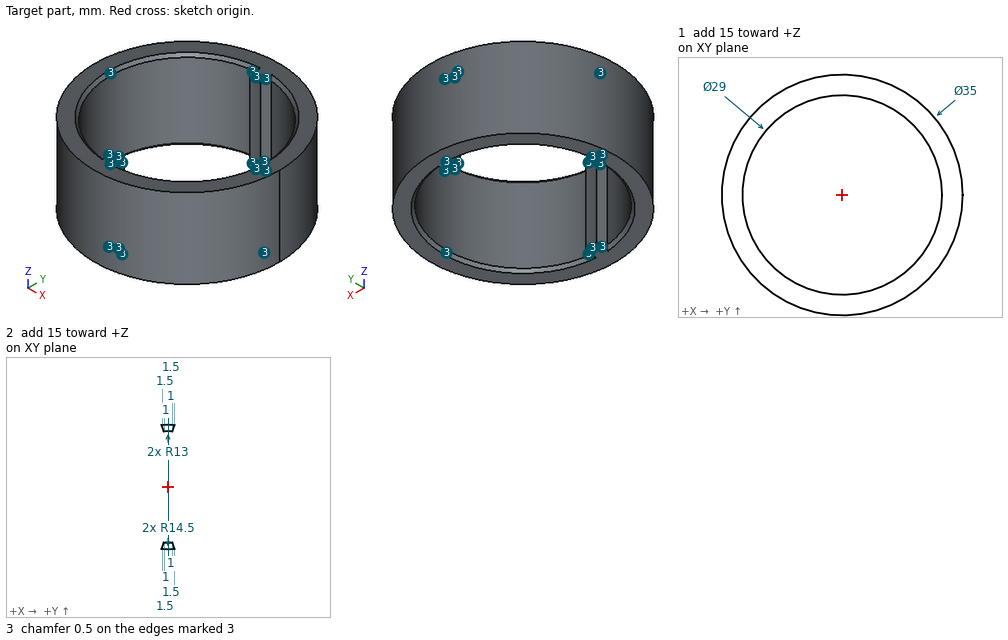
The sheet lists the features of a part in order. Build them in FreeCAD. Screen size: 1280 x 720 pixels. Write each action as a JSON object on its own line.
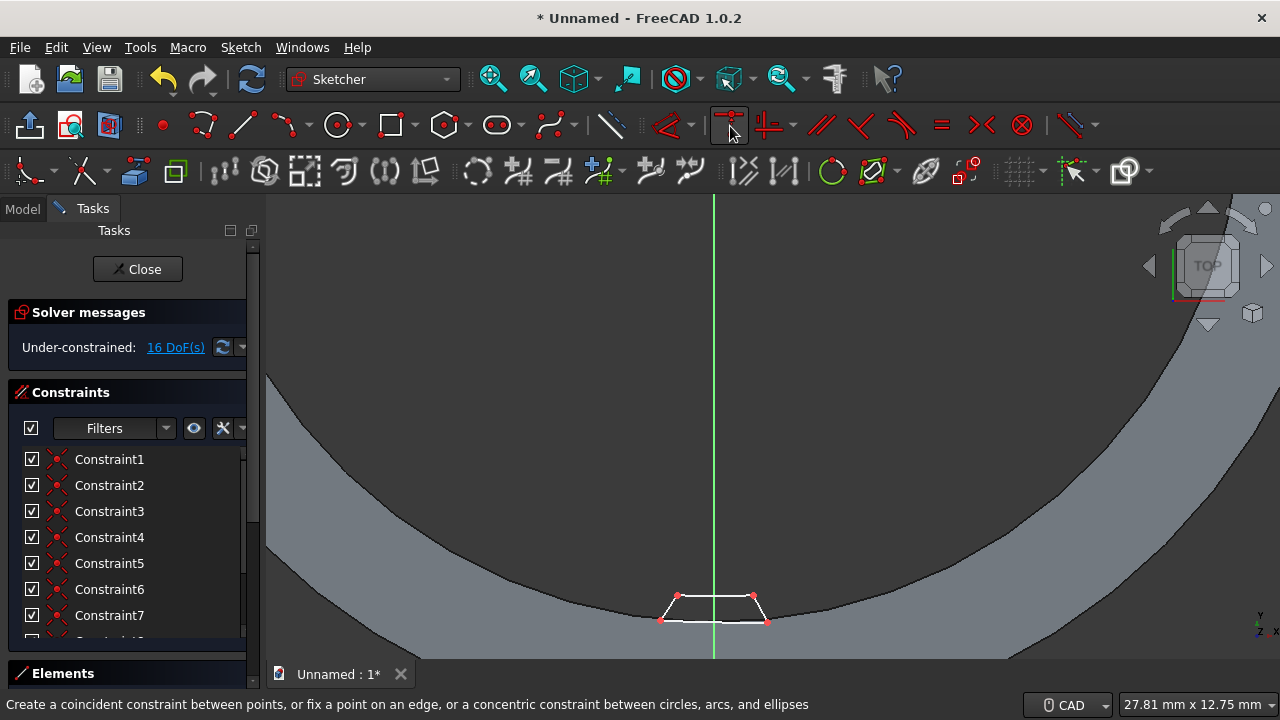
{"action": "scroll", "coordinate": [700, 570], "scroll_direction": "down", "scroll_amount": 6}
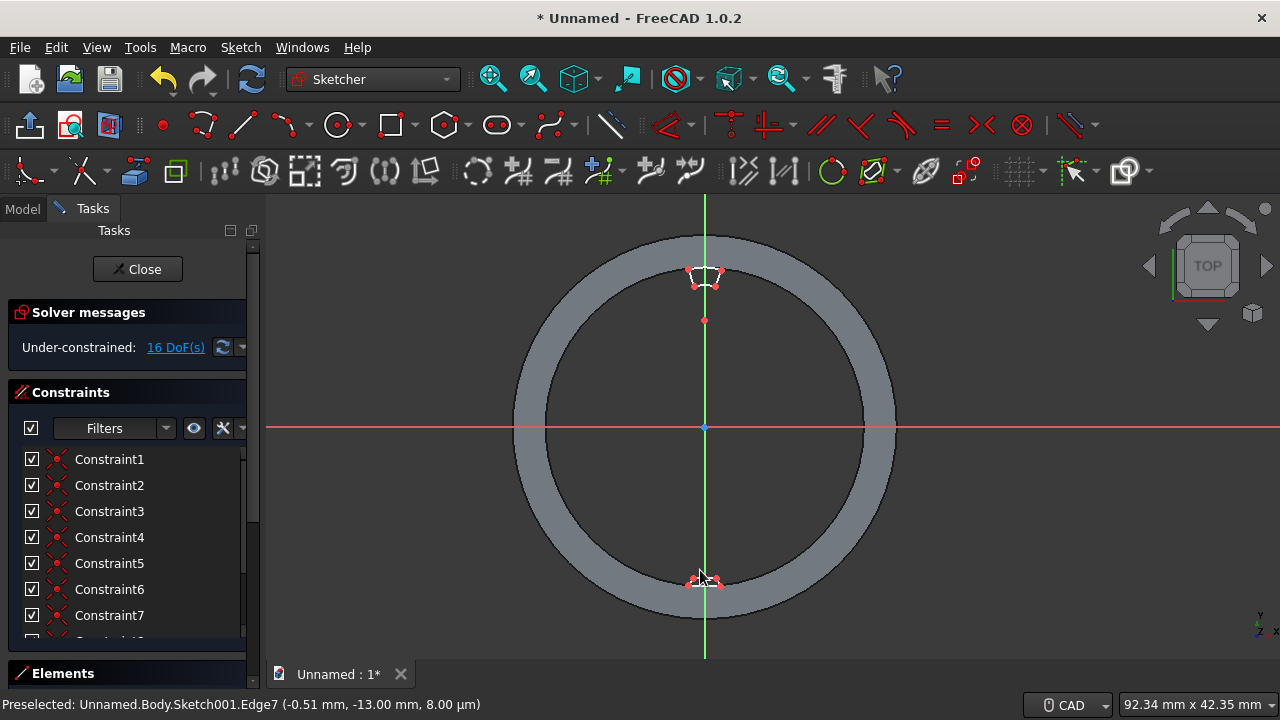
{"action": "scroll", "coordinate": [709, 285], "scroll_direction": "up", "scroll_amount": 6}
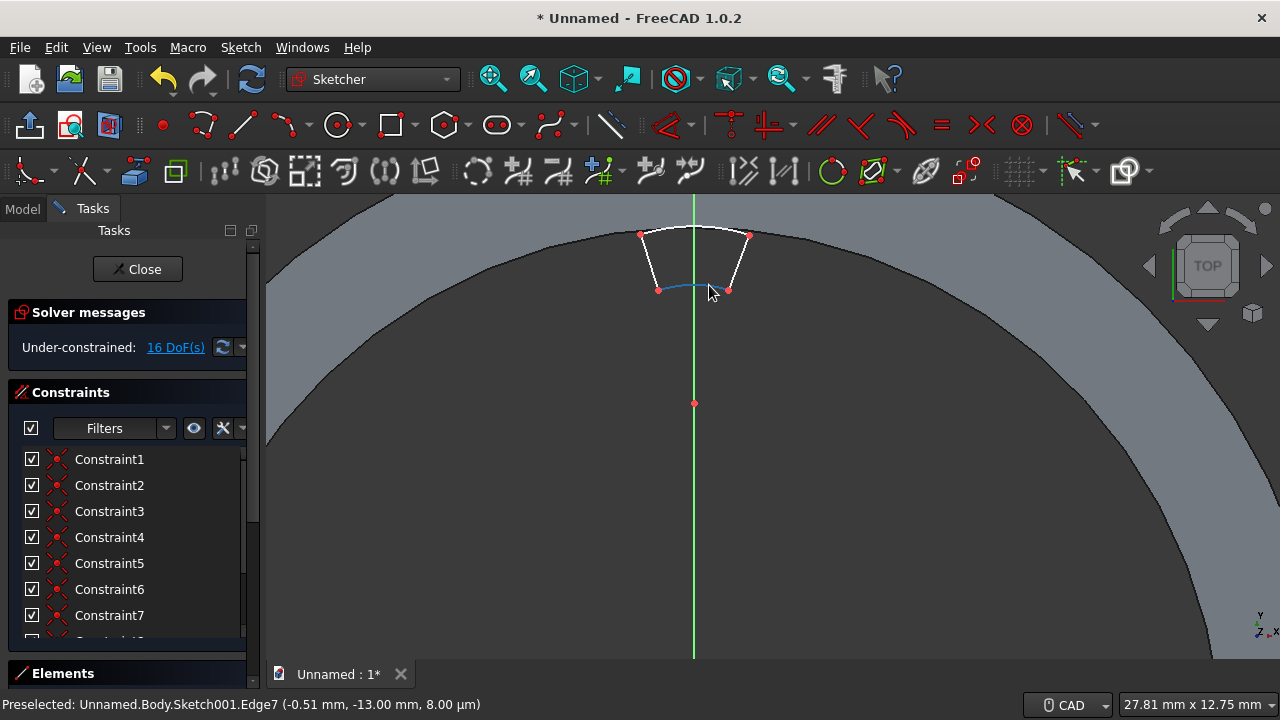
{"action": "left_click", "coordinate": [708, 286]}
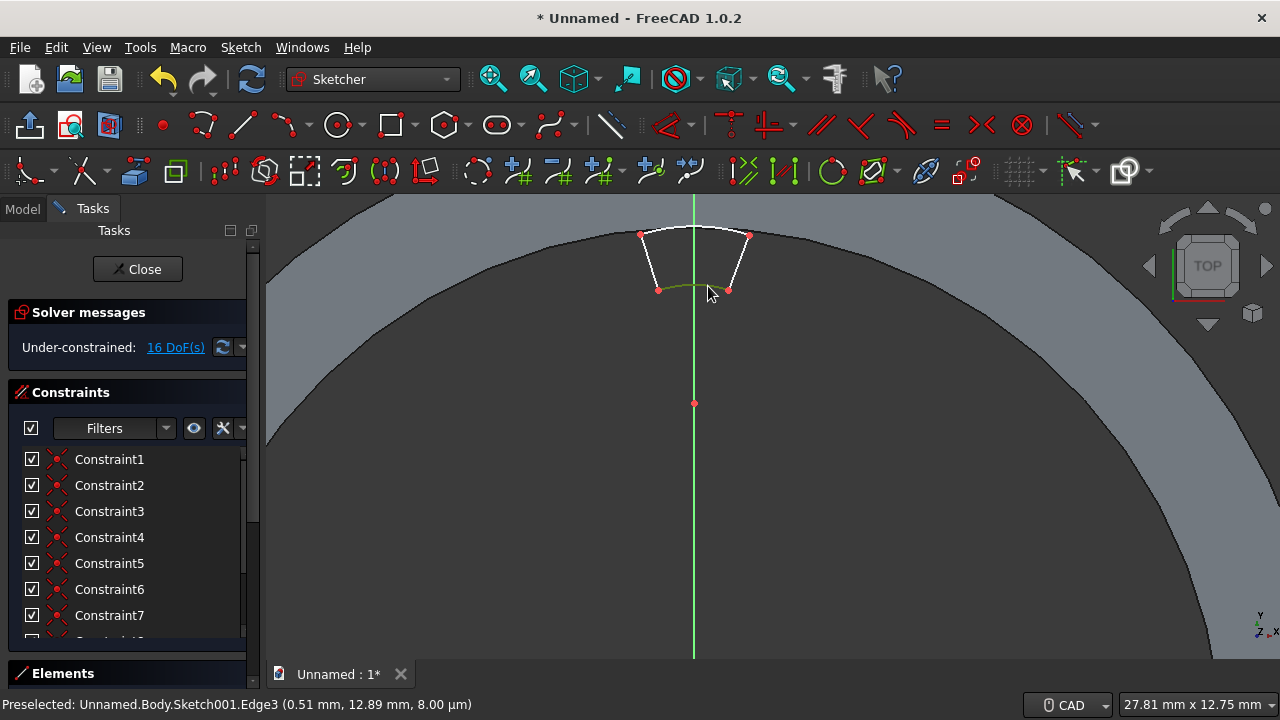
{"action": "scroll", "coordinate": [709, 284], "scroll_direction": "down", "scroll_amount": 6}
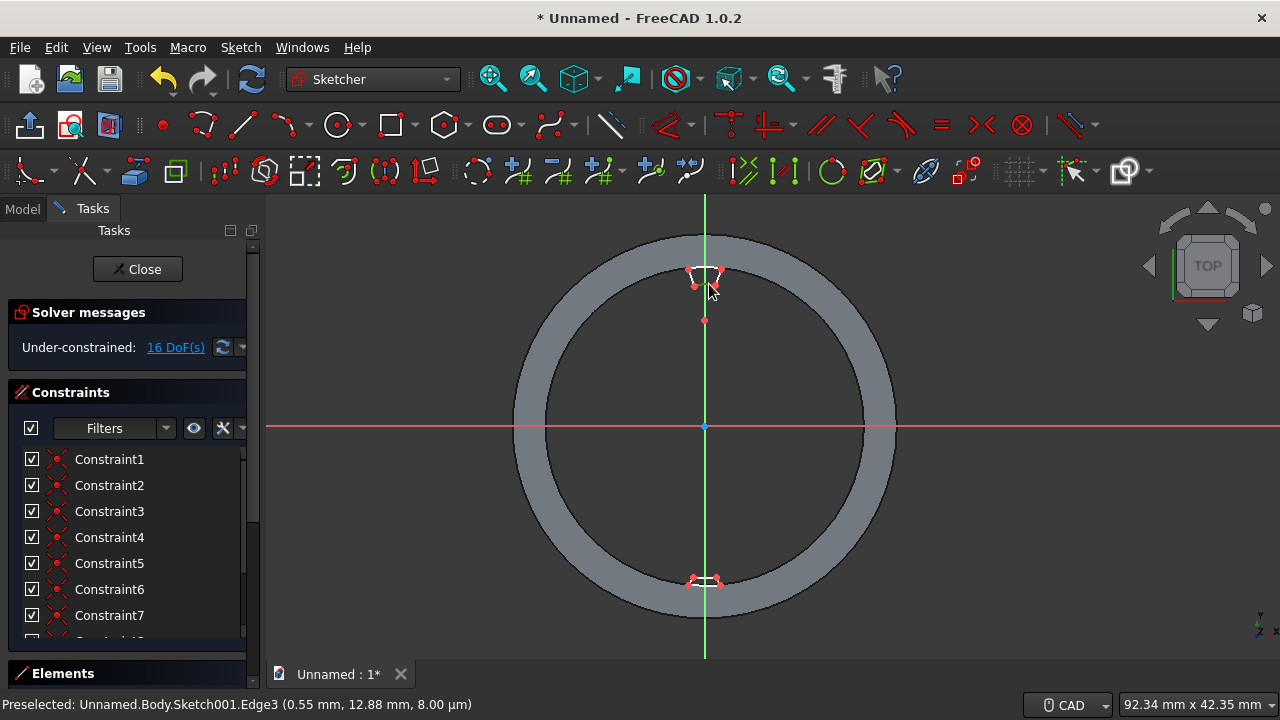
{"action": "scroll", "coordinate": [698, 585], "scroll_direction": "up", "scroll_amount": 4}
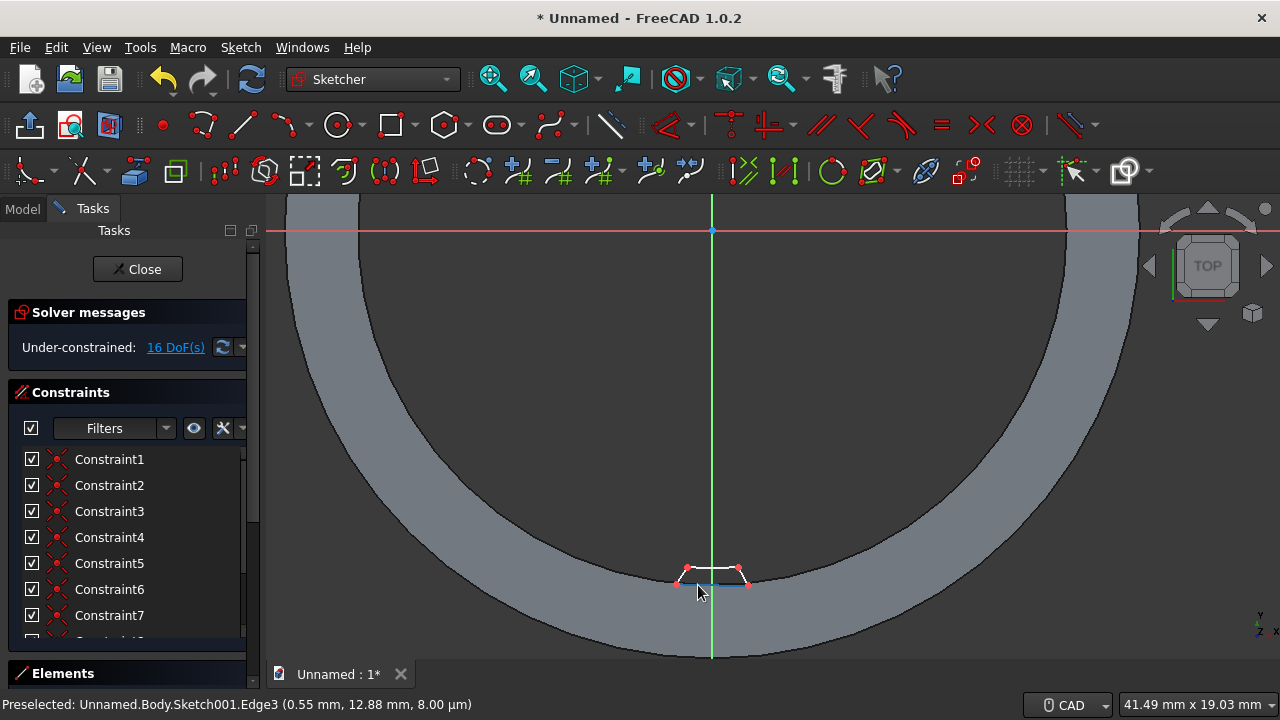
{"action": "left_click", "coordinate": [698, 585]}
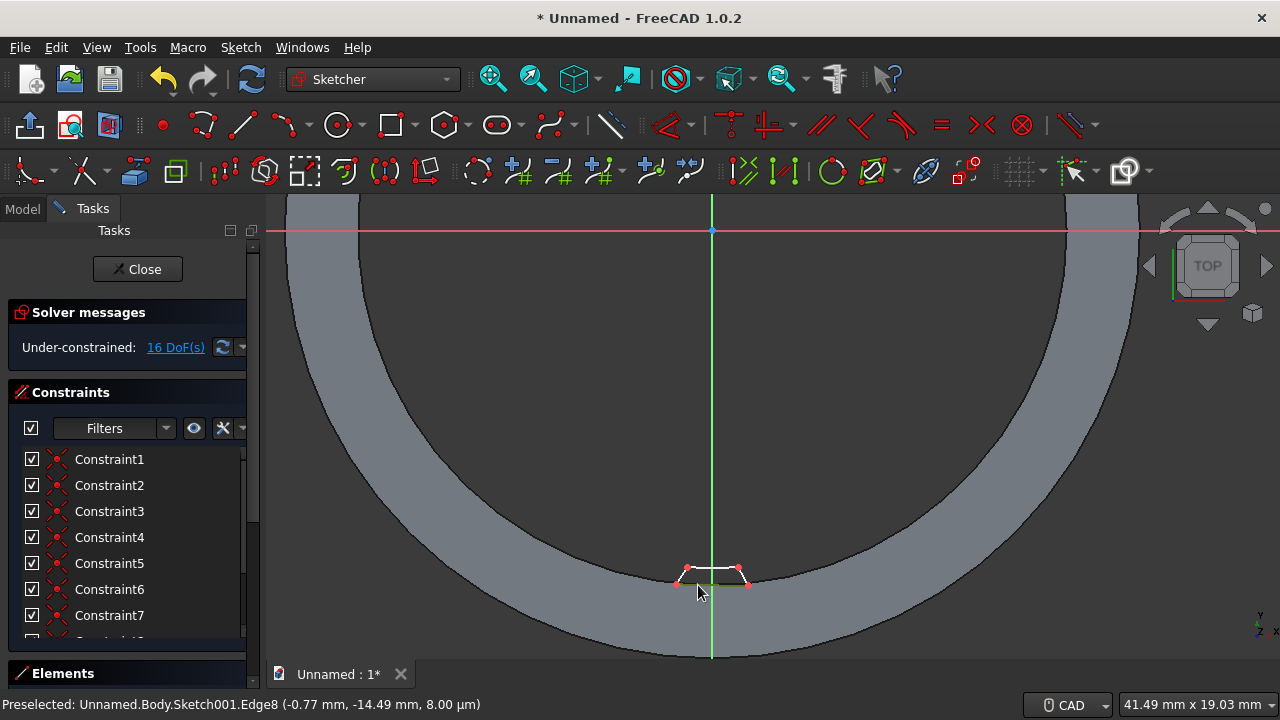
{"action": "left_click", "coordinate": [730, 126]}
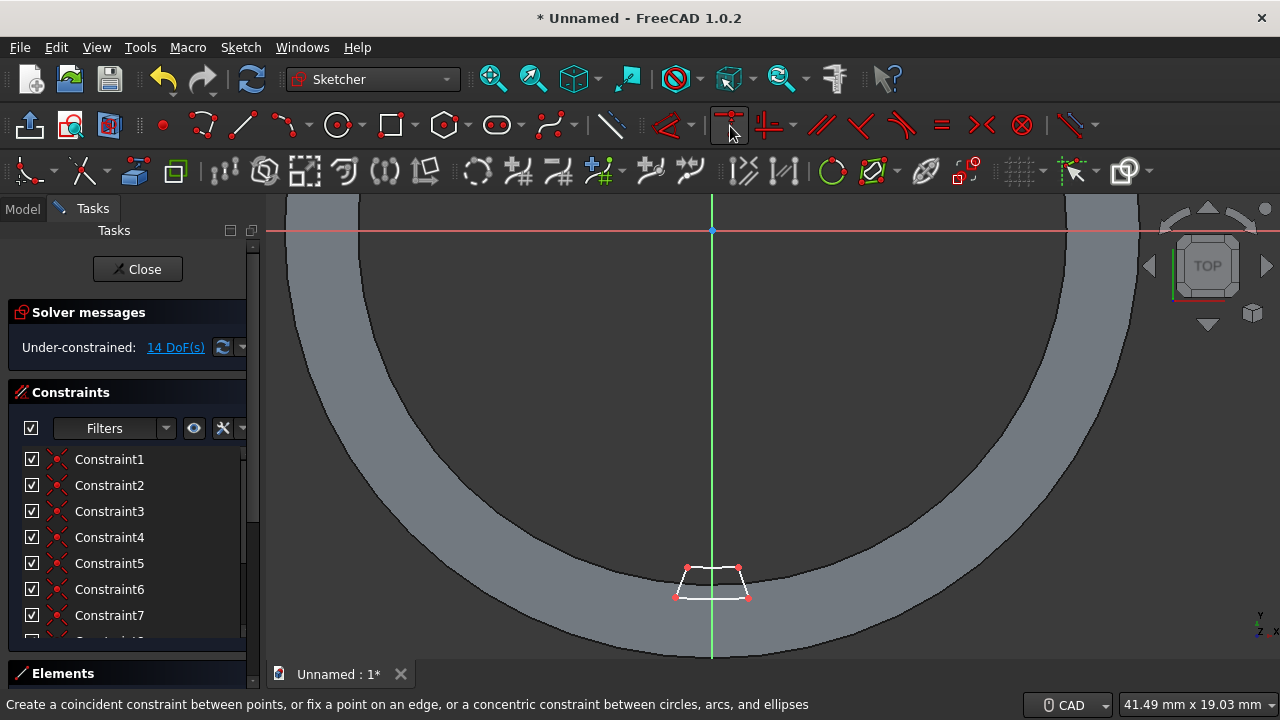
{"action": "scroll", "coordinate": [698, 586], "scroll_direction": "down", "scroll_amount": 4}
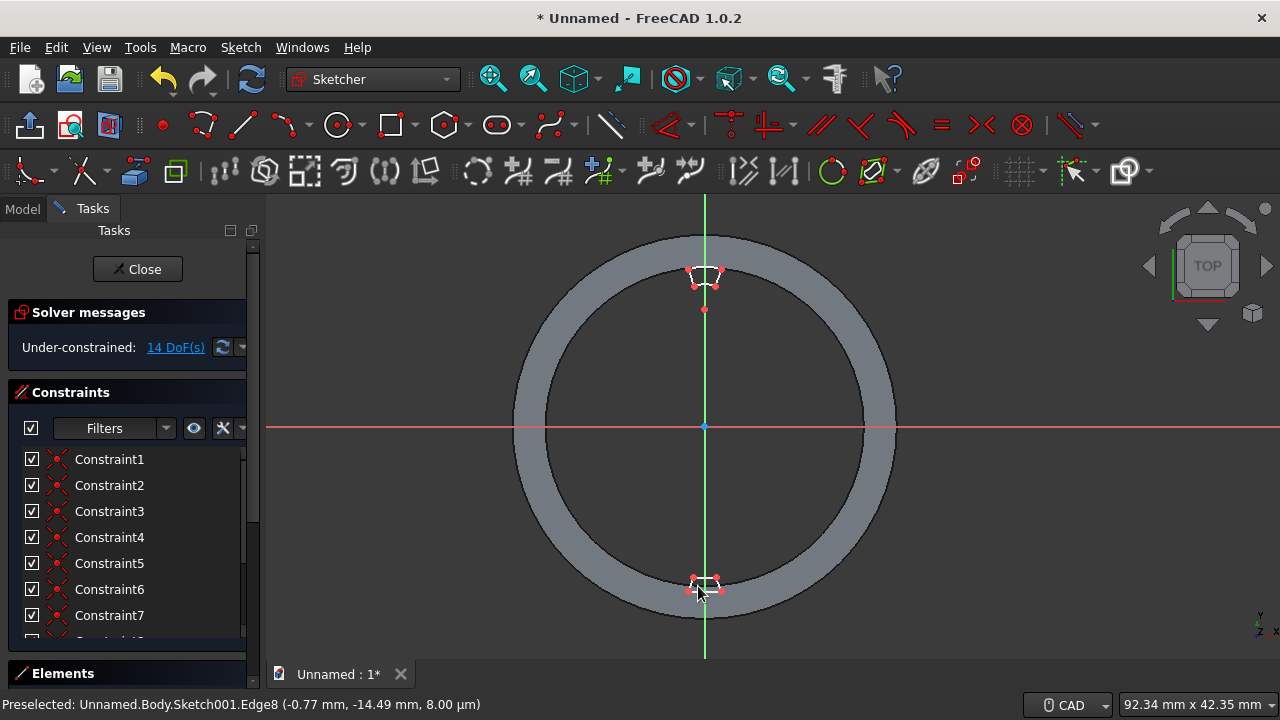
{"action": "scroll", "coordinate": [705, 368], "scroll_direction": "up", "scroll_amount": 3}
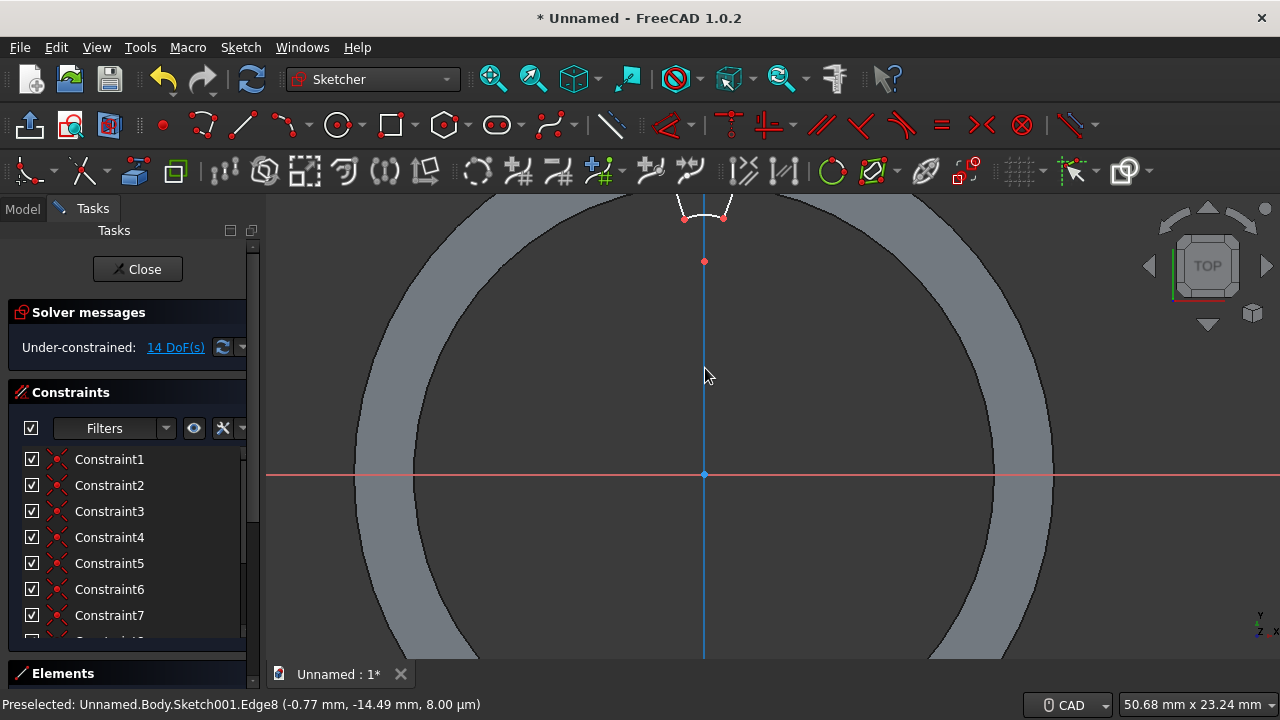
{"action": "left_click_drag", "start_coordinate": [694, 251], "coordinate": [714, 485]}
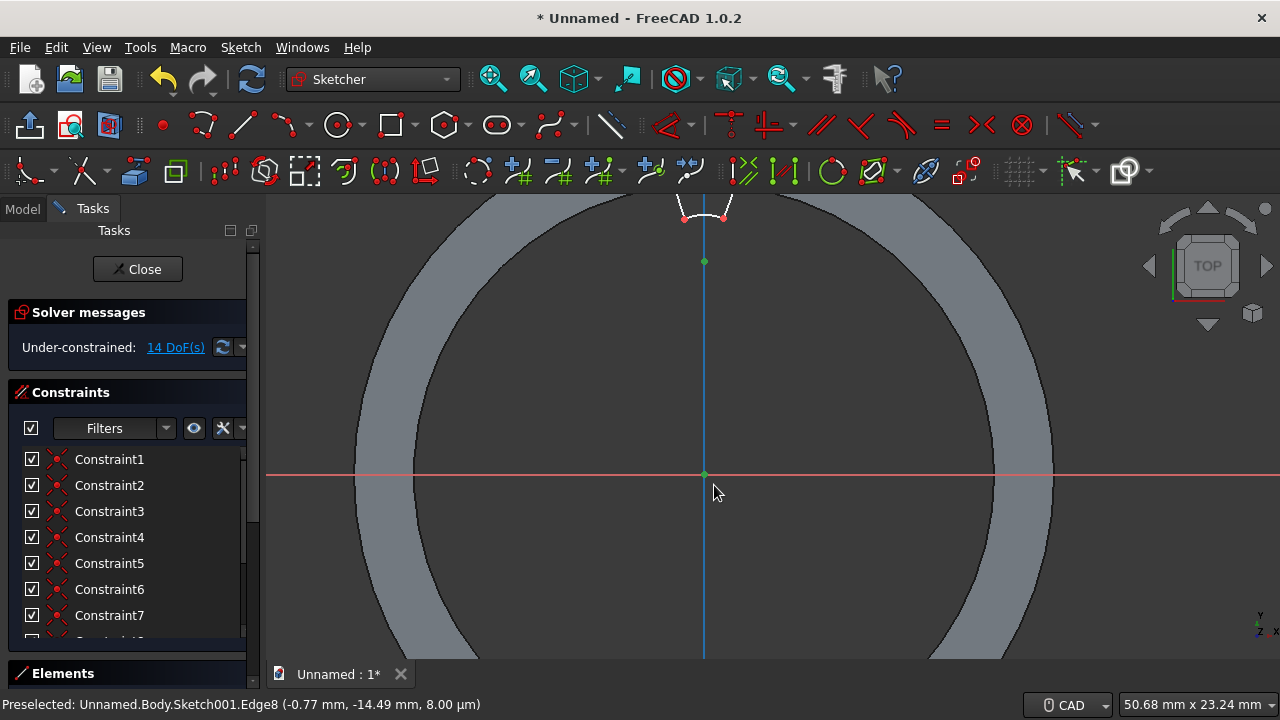
{"action": "left_click", "coordinate": [730, 126]}